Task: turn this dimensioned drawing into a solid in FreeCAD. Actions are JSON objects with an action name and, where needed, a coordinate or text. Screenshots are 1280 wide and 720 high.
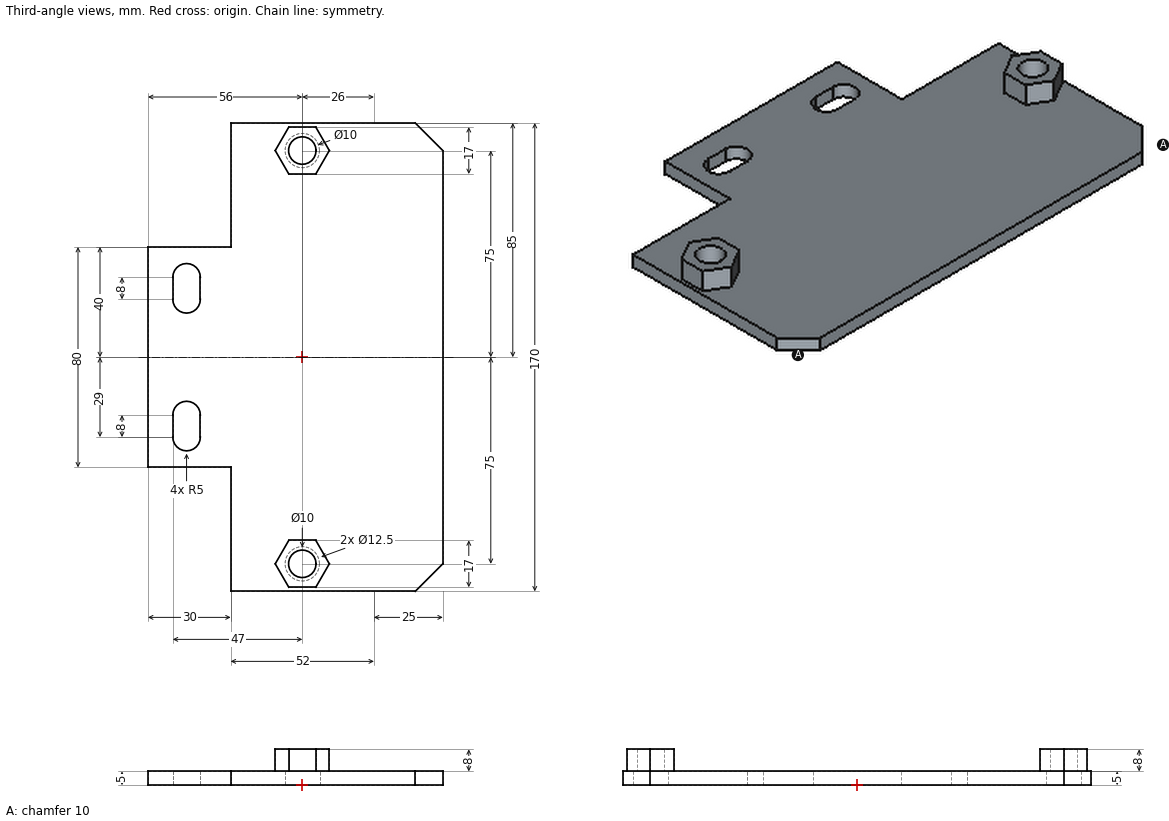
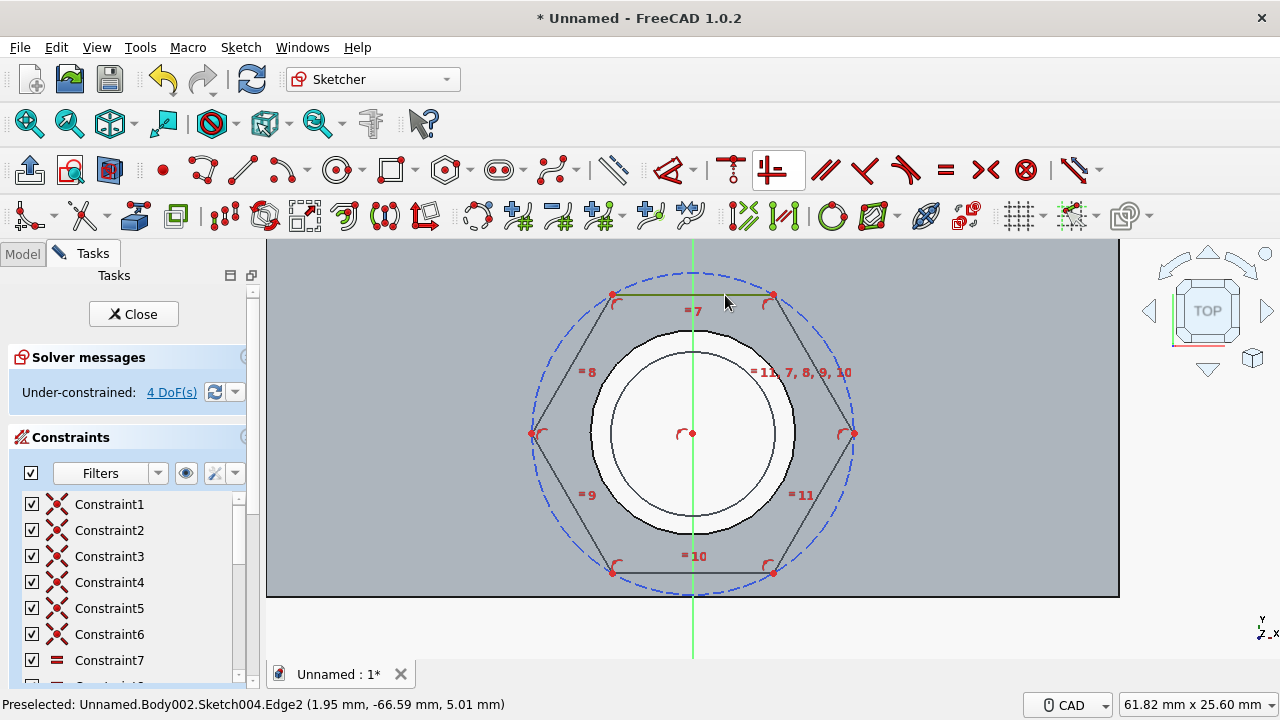
{"action": "left_click", "coordinate": [800, 170]}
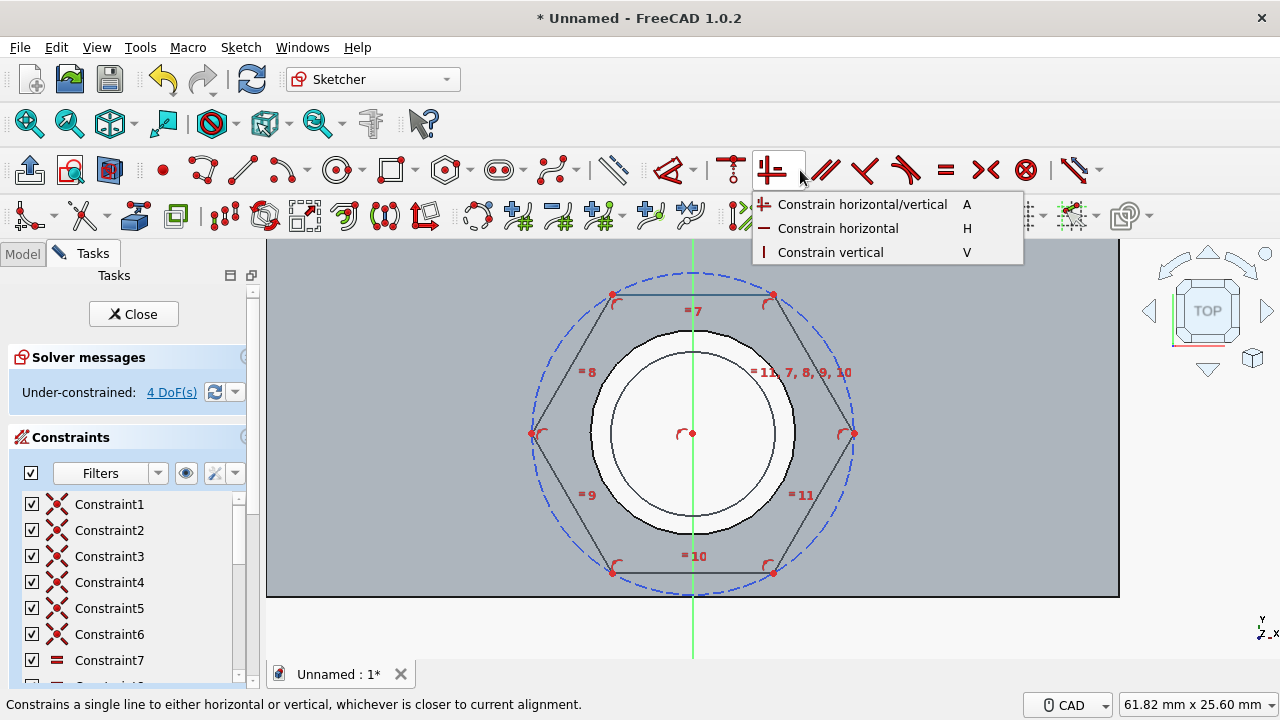
{"action": "left_click", "coordinate": [888, 228]}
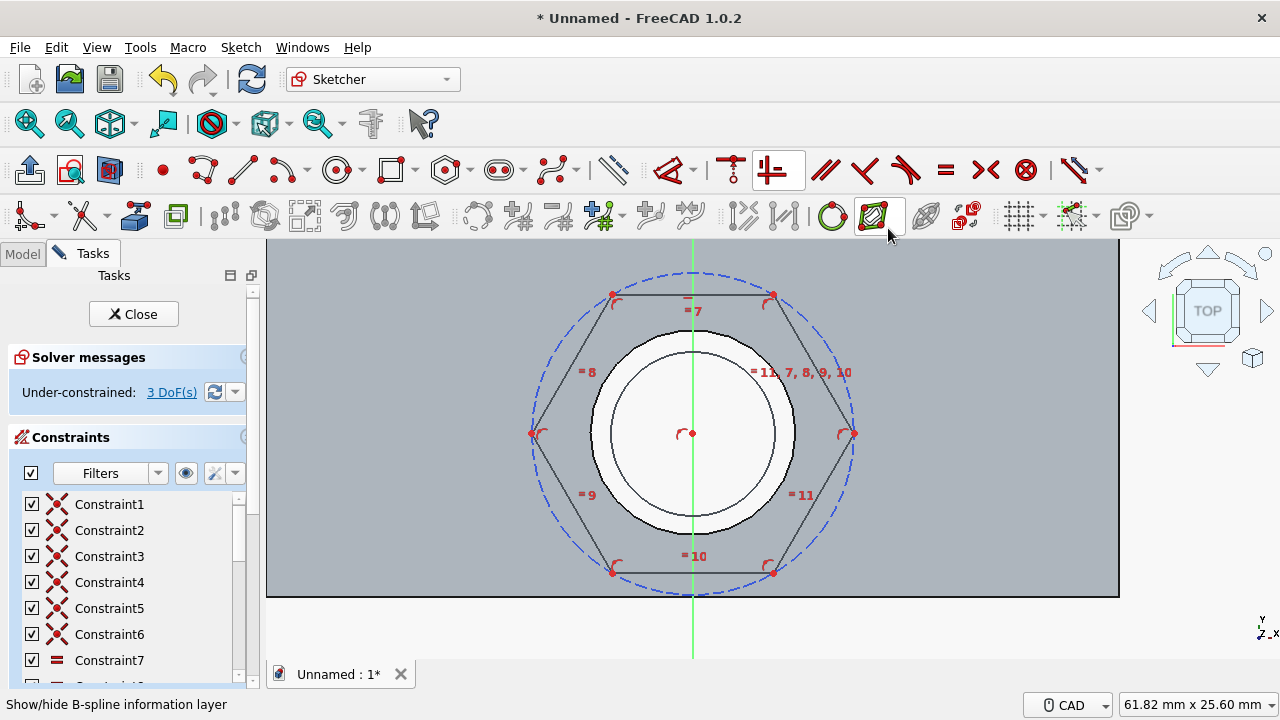
{"action": "left_click", "coordinate": [668, 170]}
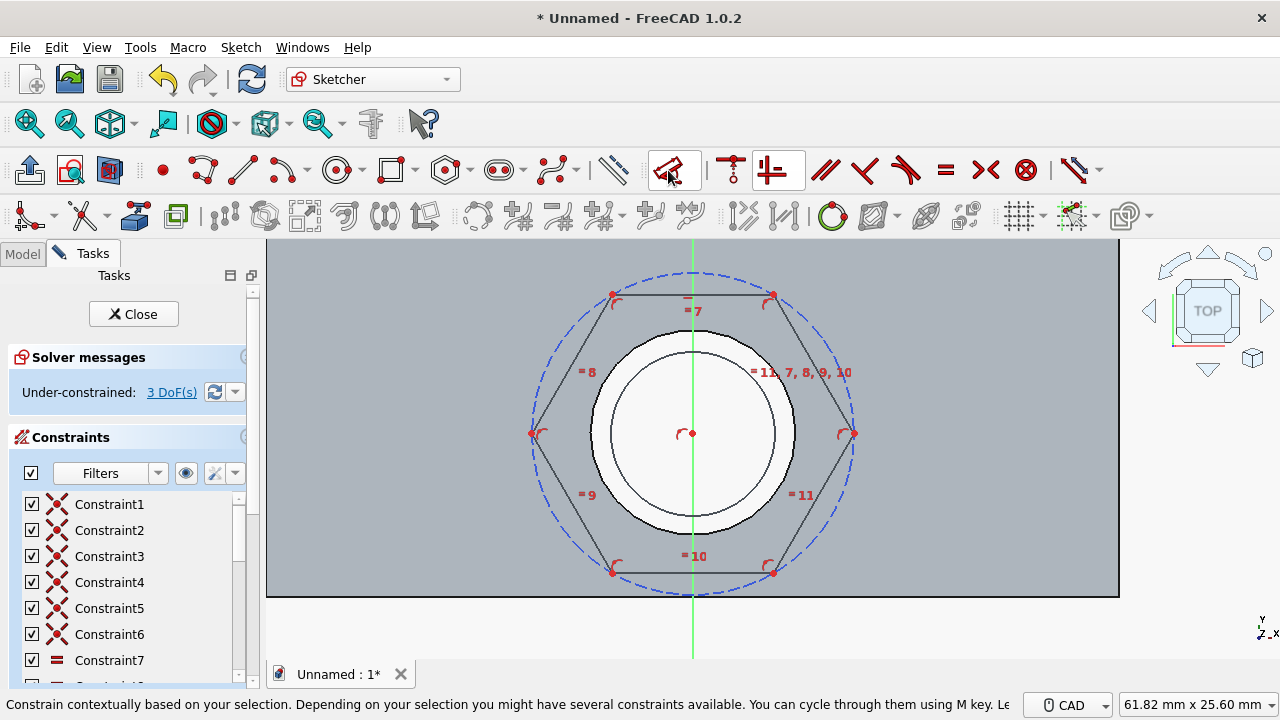
{"action": "left_click", "coordinate": [751, 376]}
{"action": "left_click", "coordinate": [774, 353]}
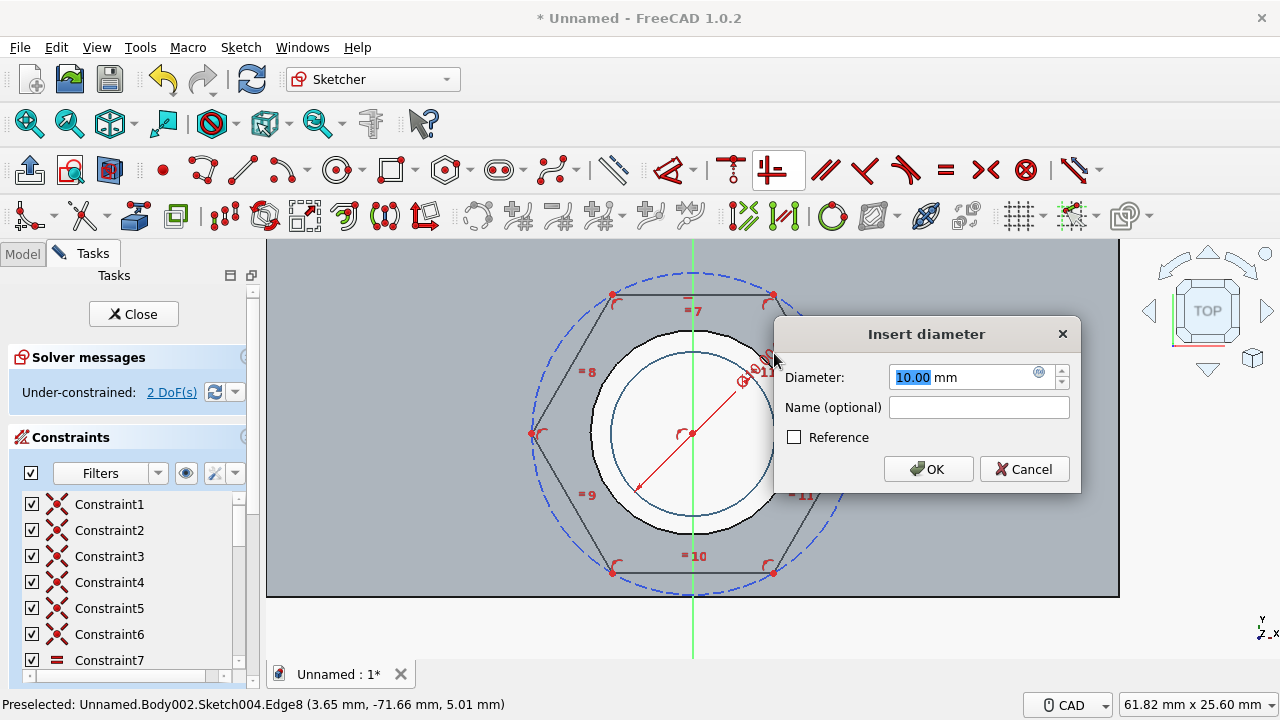
{"action": "type", "text": "10"}
{"action": "key", "text": "Return"}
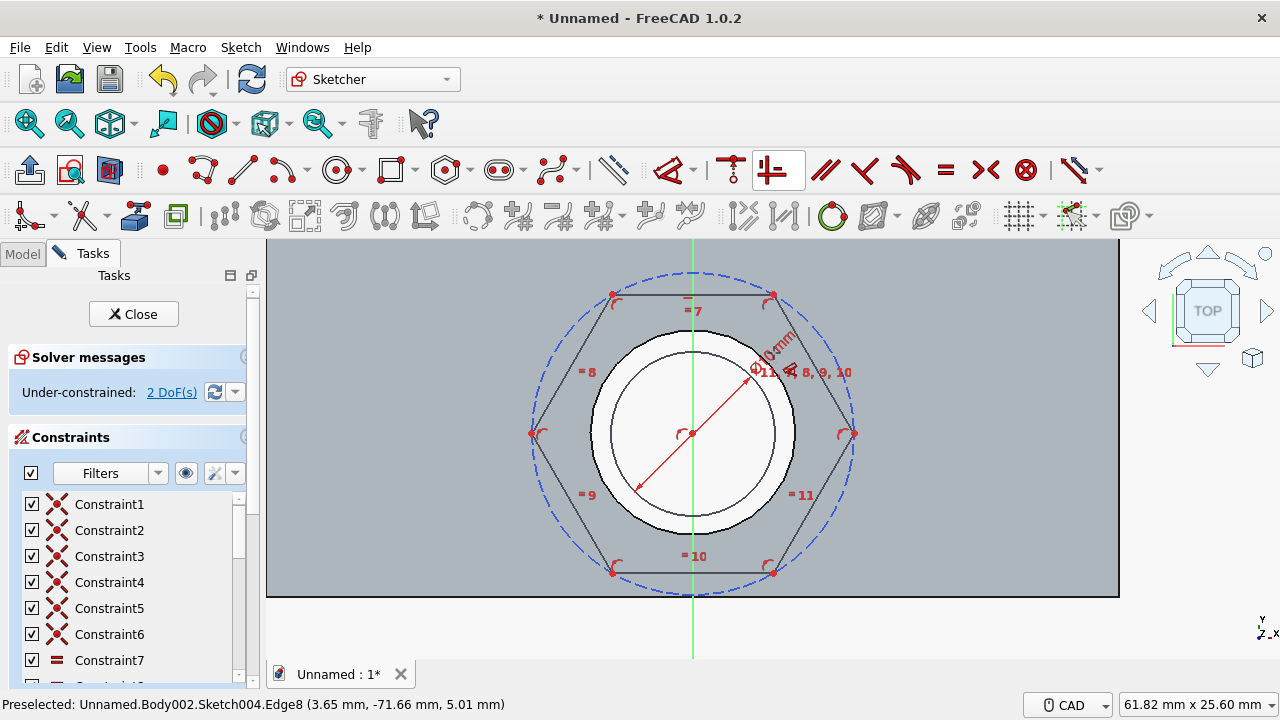
{"action": "left_click", "coordinate": [612, 573]}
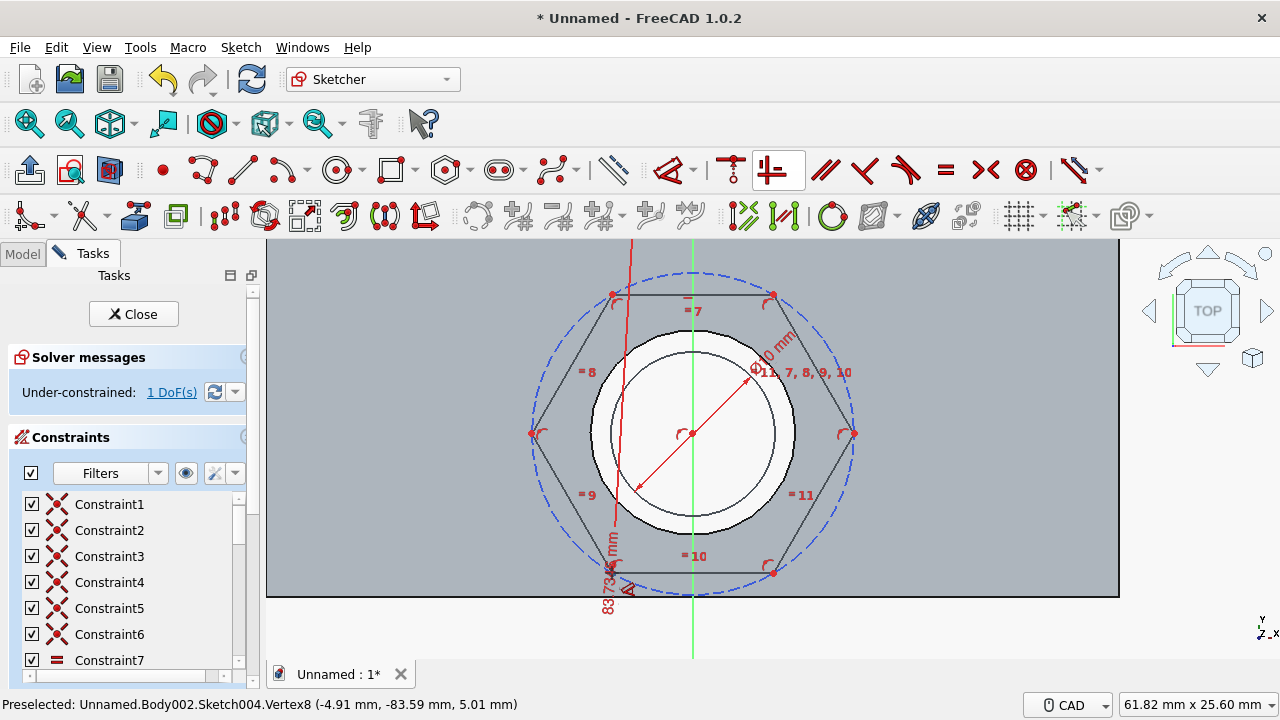
{"action": "left_click", "coordinate": [773, 295]}
{"action": "left_click", "coordinate": [578, 434]}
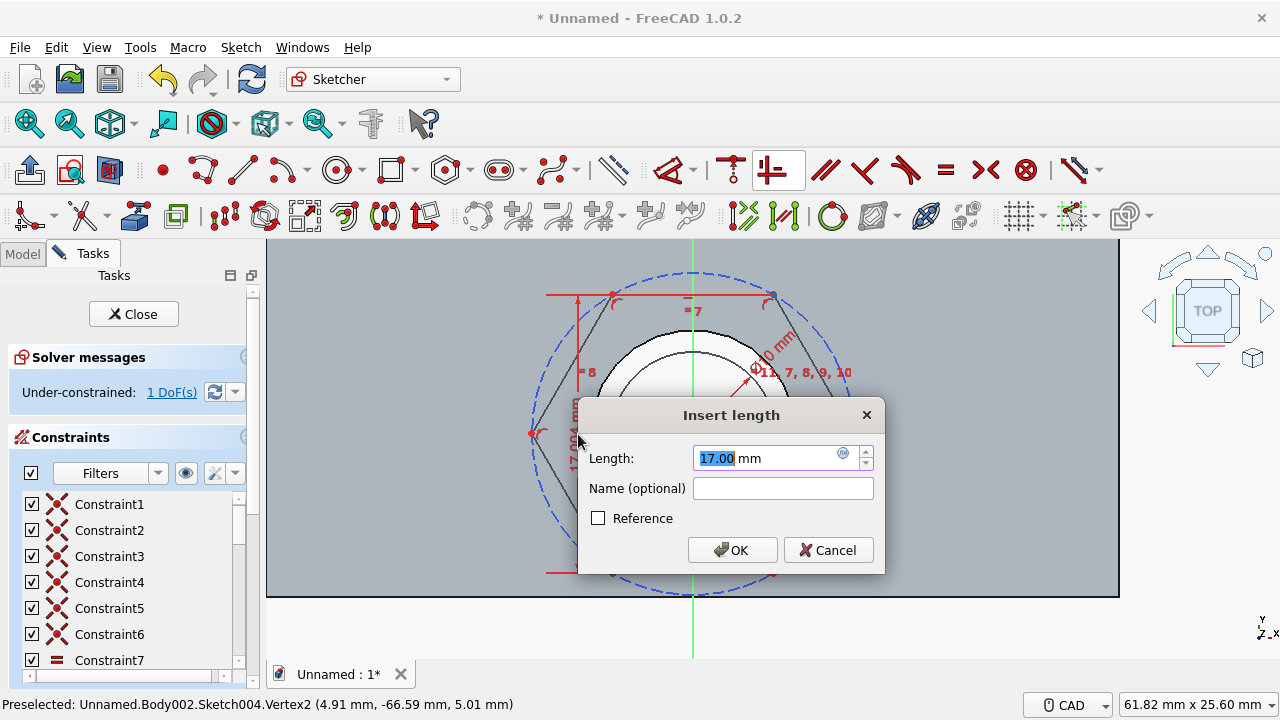
{"action": "type", "text": "17"}
{"action": "key", "text": "Return"}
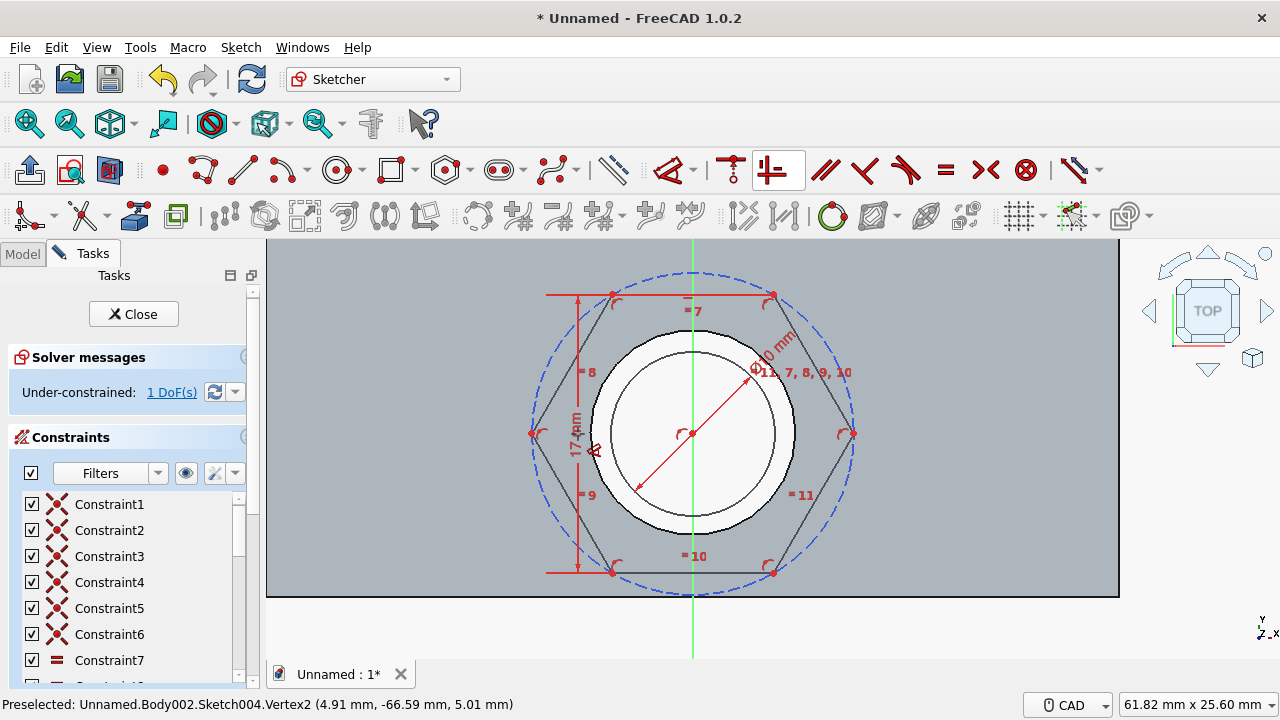
{"action": "left_click", "coordinate": [693, 434]}
{"action": "left_click", "coordinate": [727, 312]}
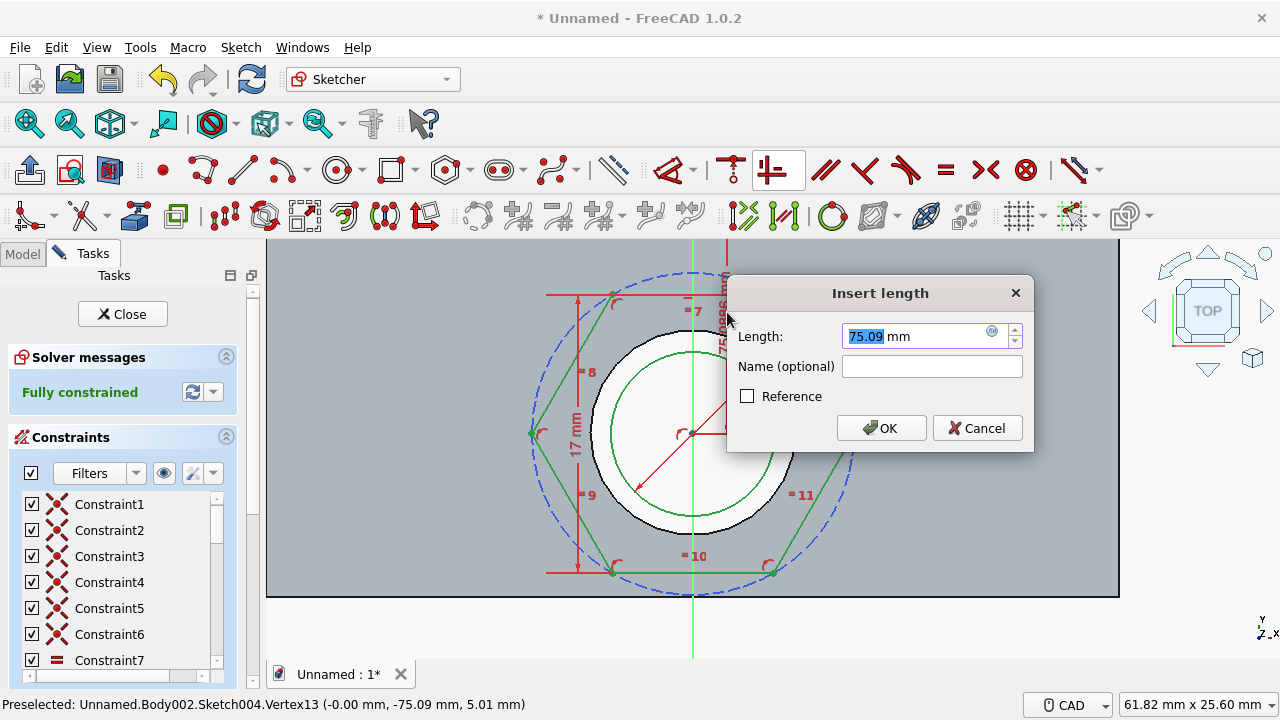
{"action": "type", "text": "75"}
{"action": "key", "text": "Return"}
{"action": "key", "text": "Escape"}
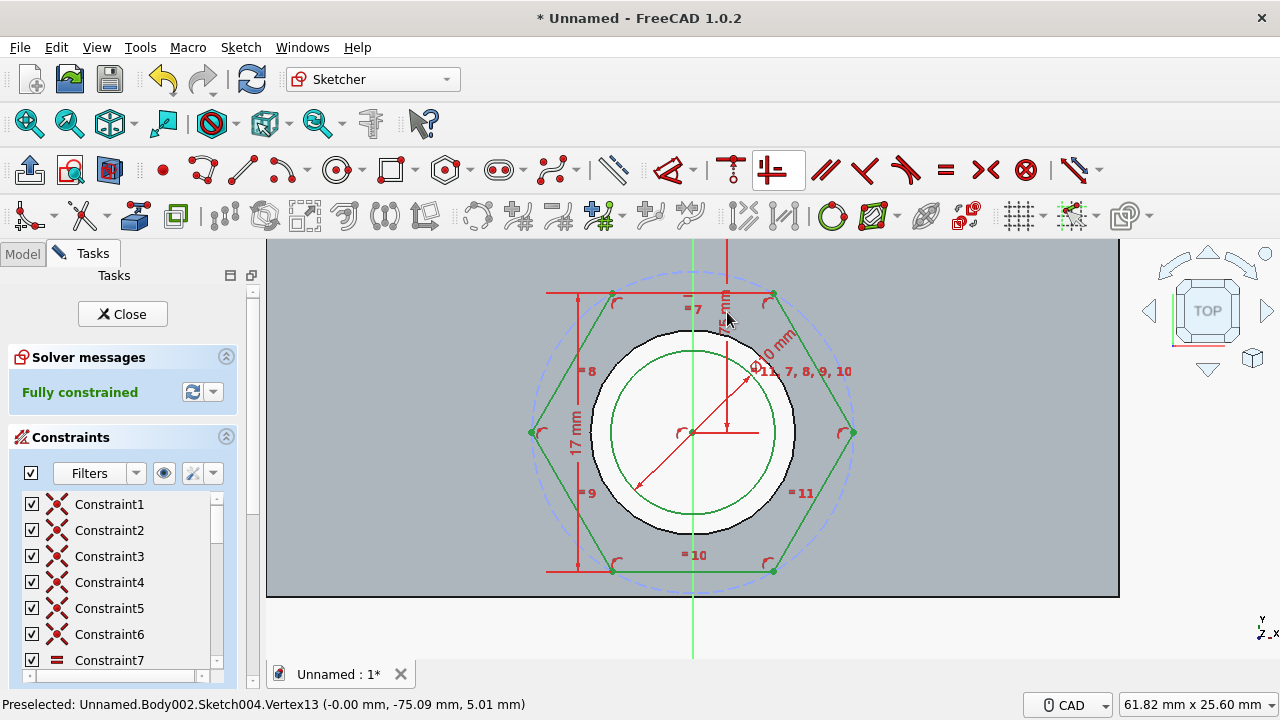
{"action": "left_click", "coordinate": [123, 314]}